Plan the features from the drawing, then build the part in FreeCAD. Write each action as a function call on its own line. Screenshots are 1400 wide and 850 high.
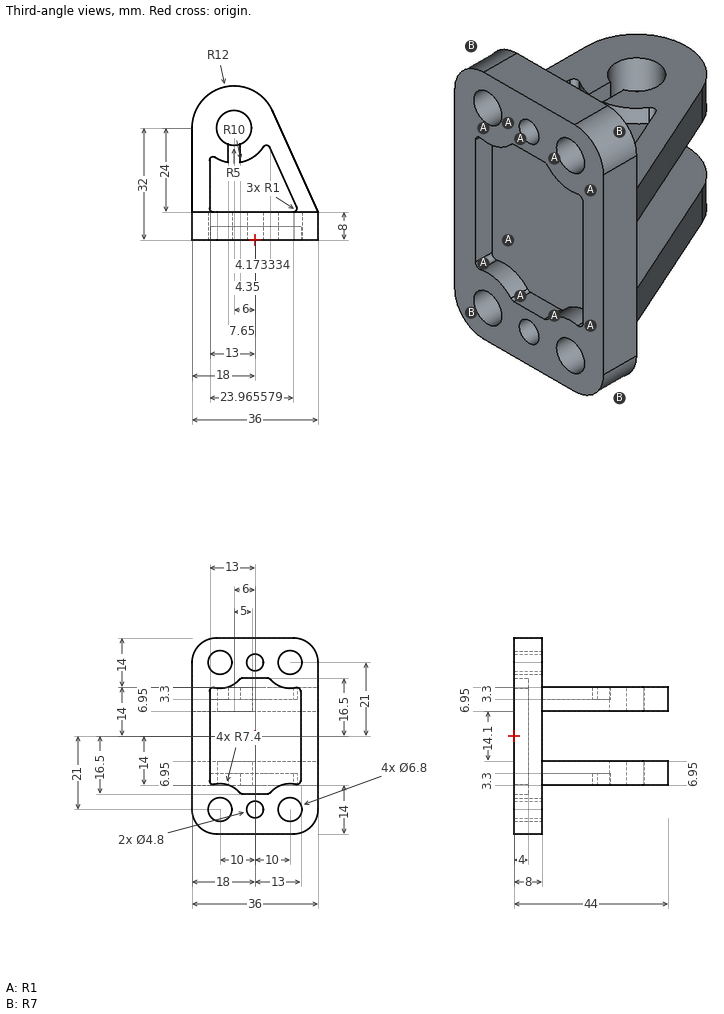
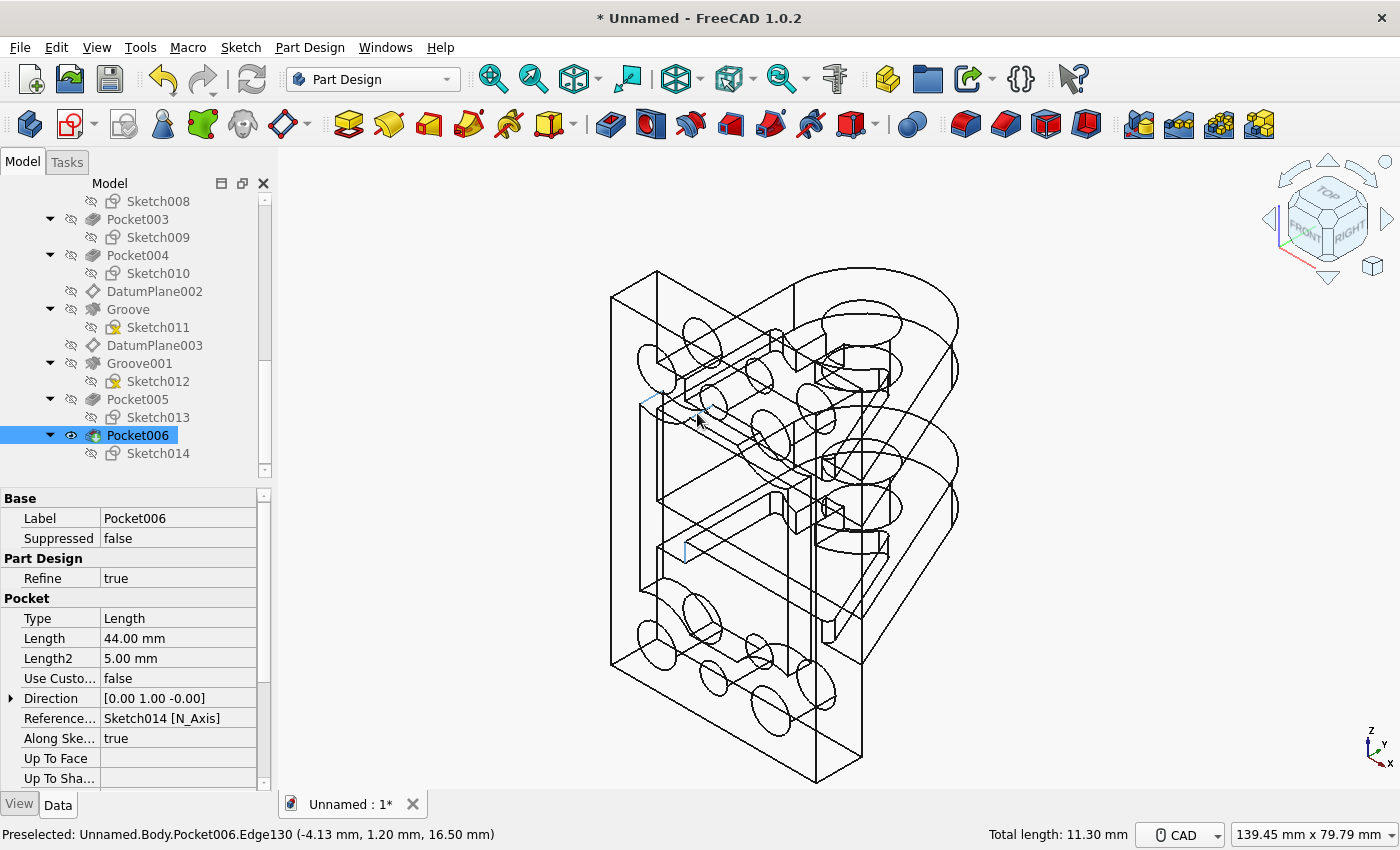
click(746, 439, ctrl)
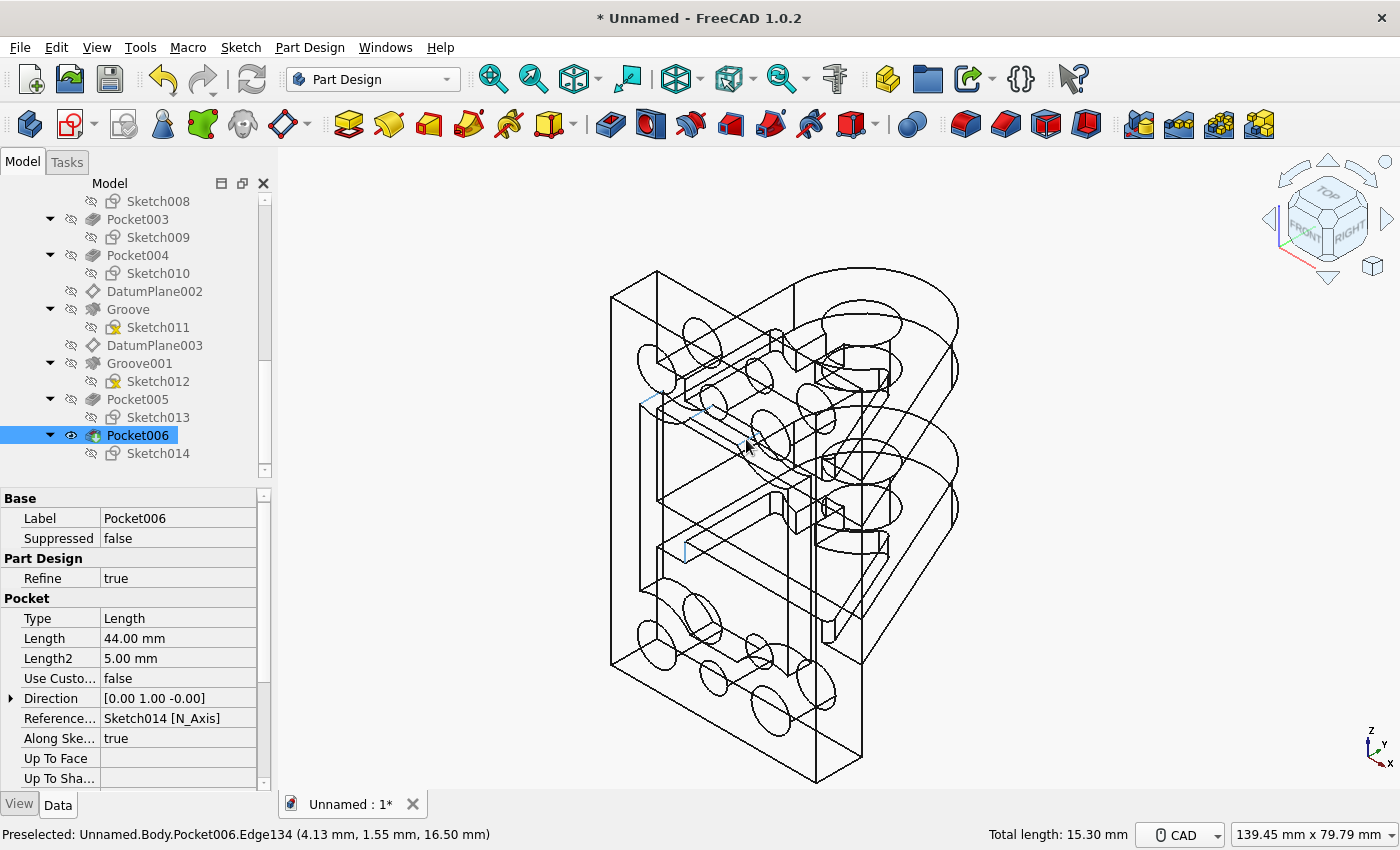
click(799, 482, ctrl)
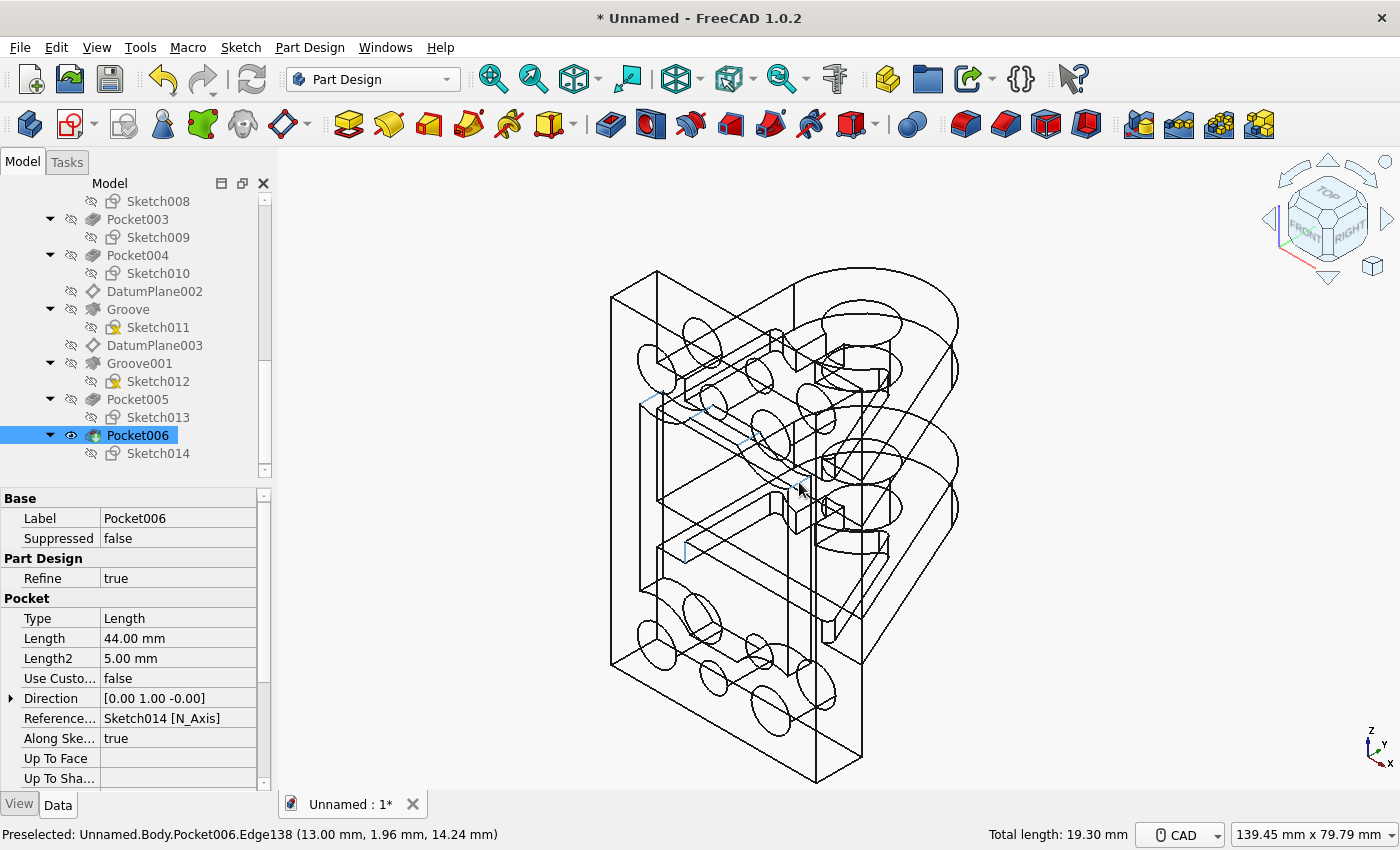
click(799, 669, ctrl)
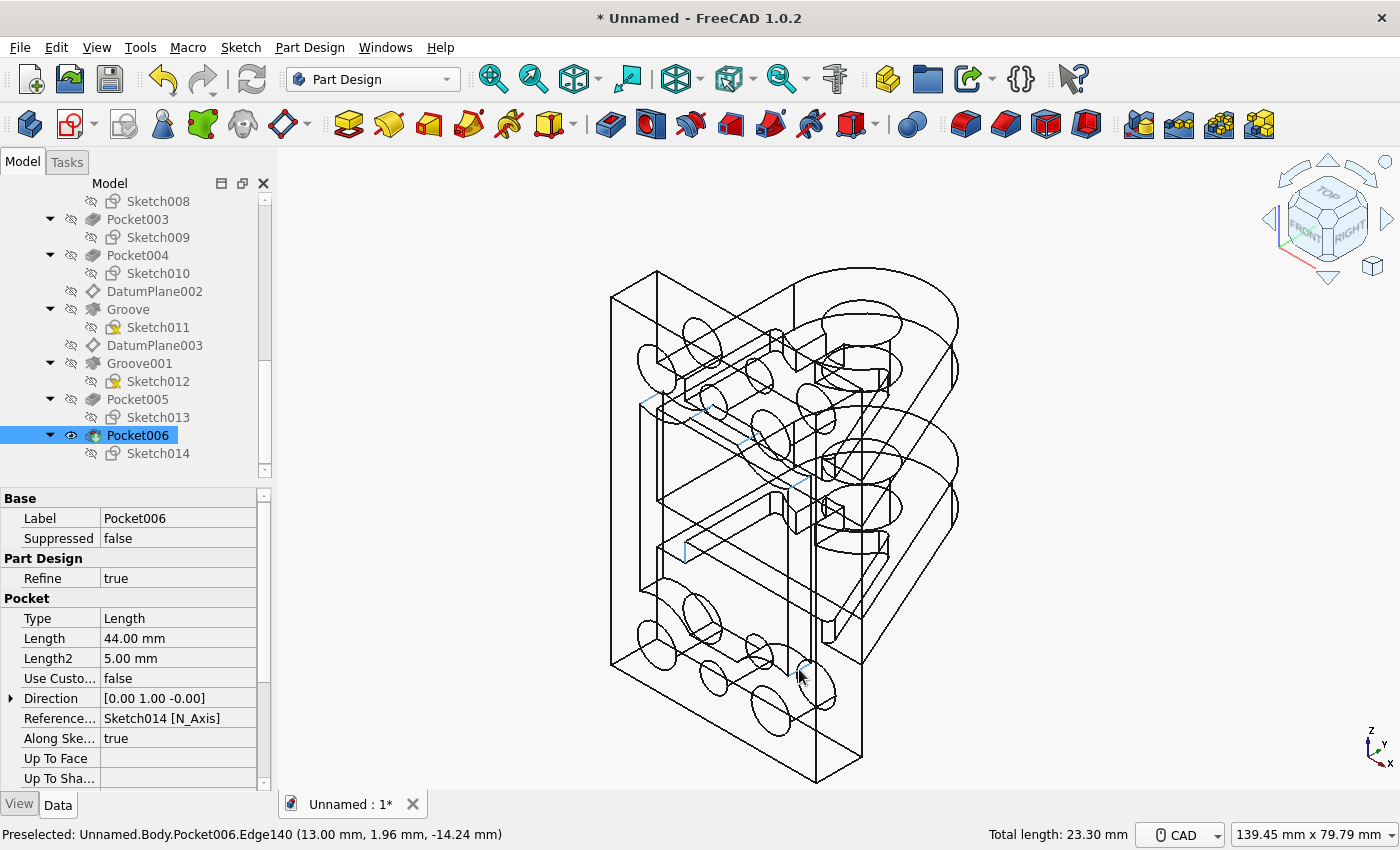
click(757, 650, ctrl)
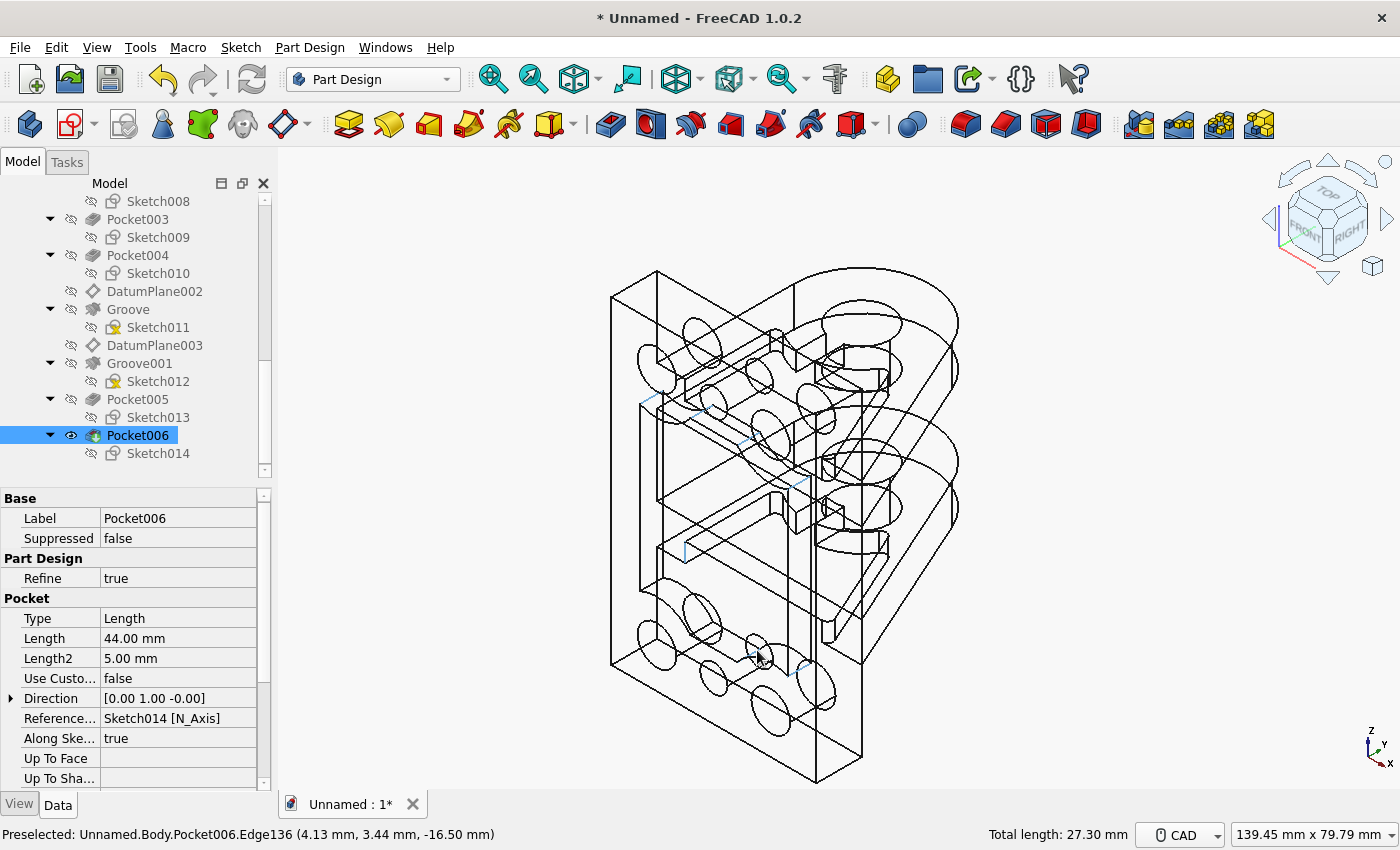
click(702, 628, ctrl)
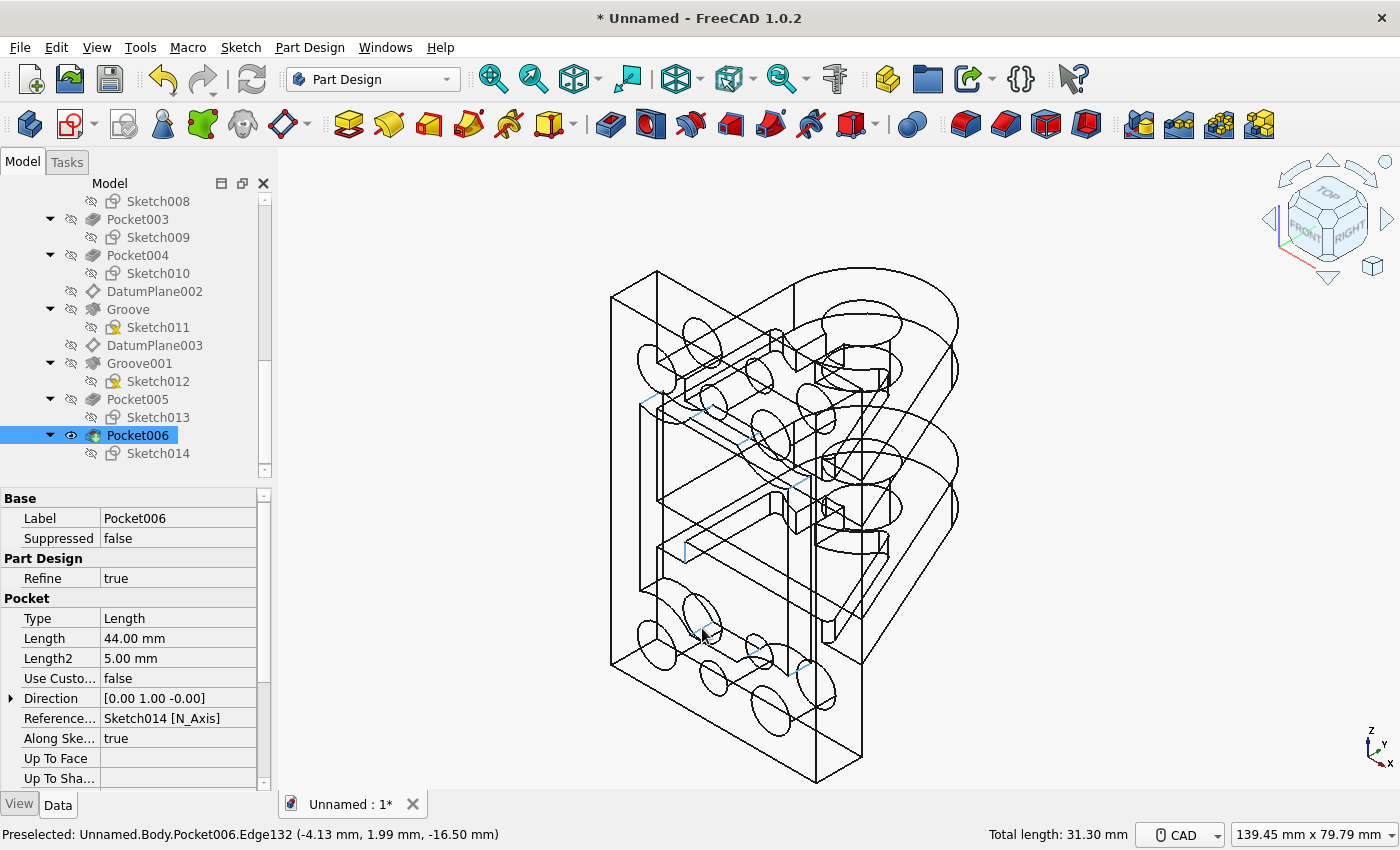
click(651, 583, ctrl)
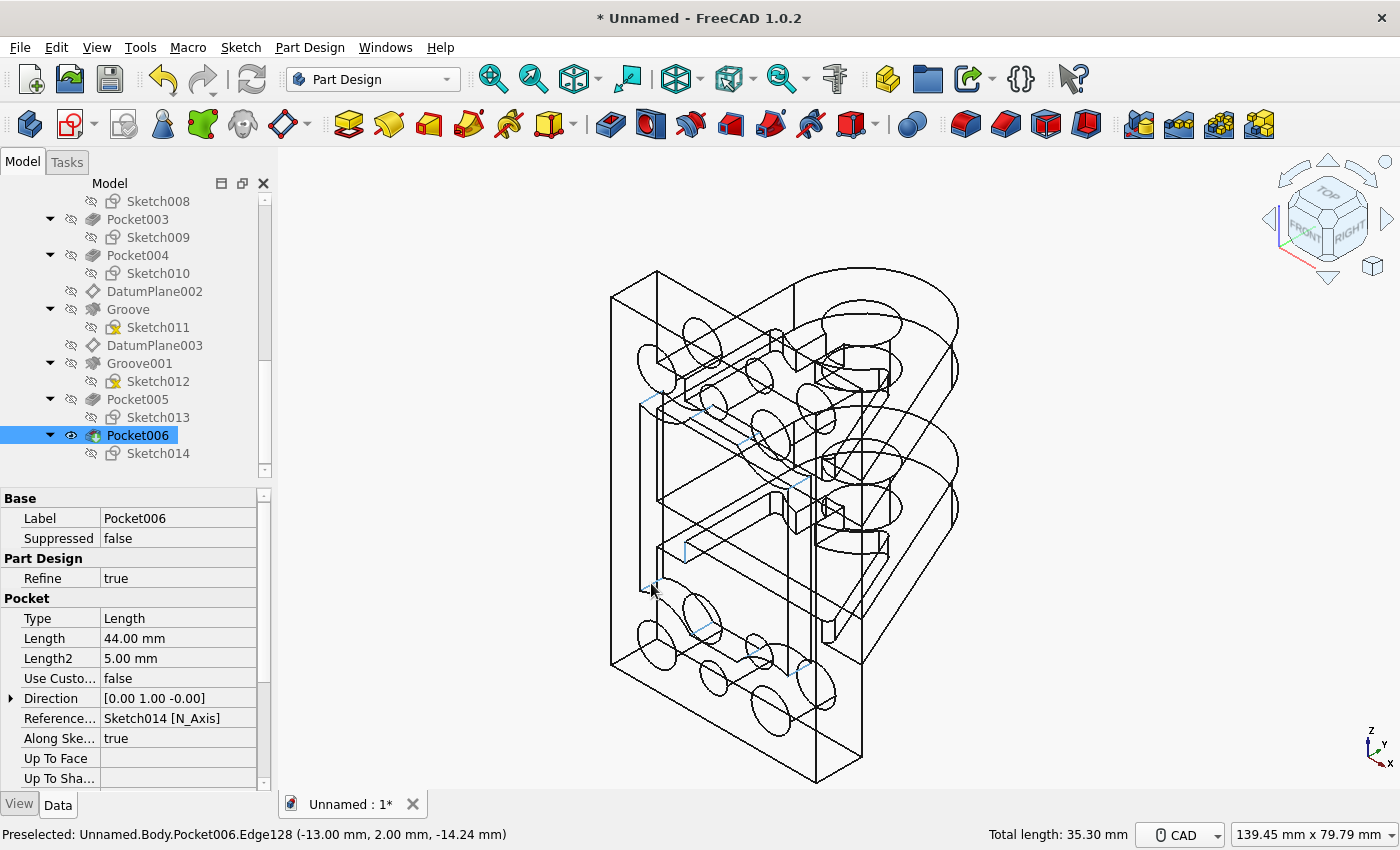
click(685, 389, ctrl)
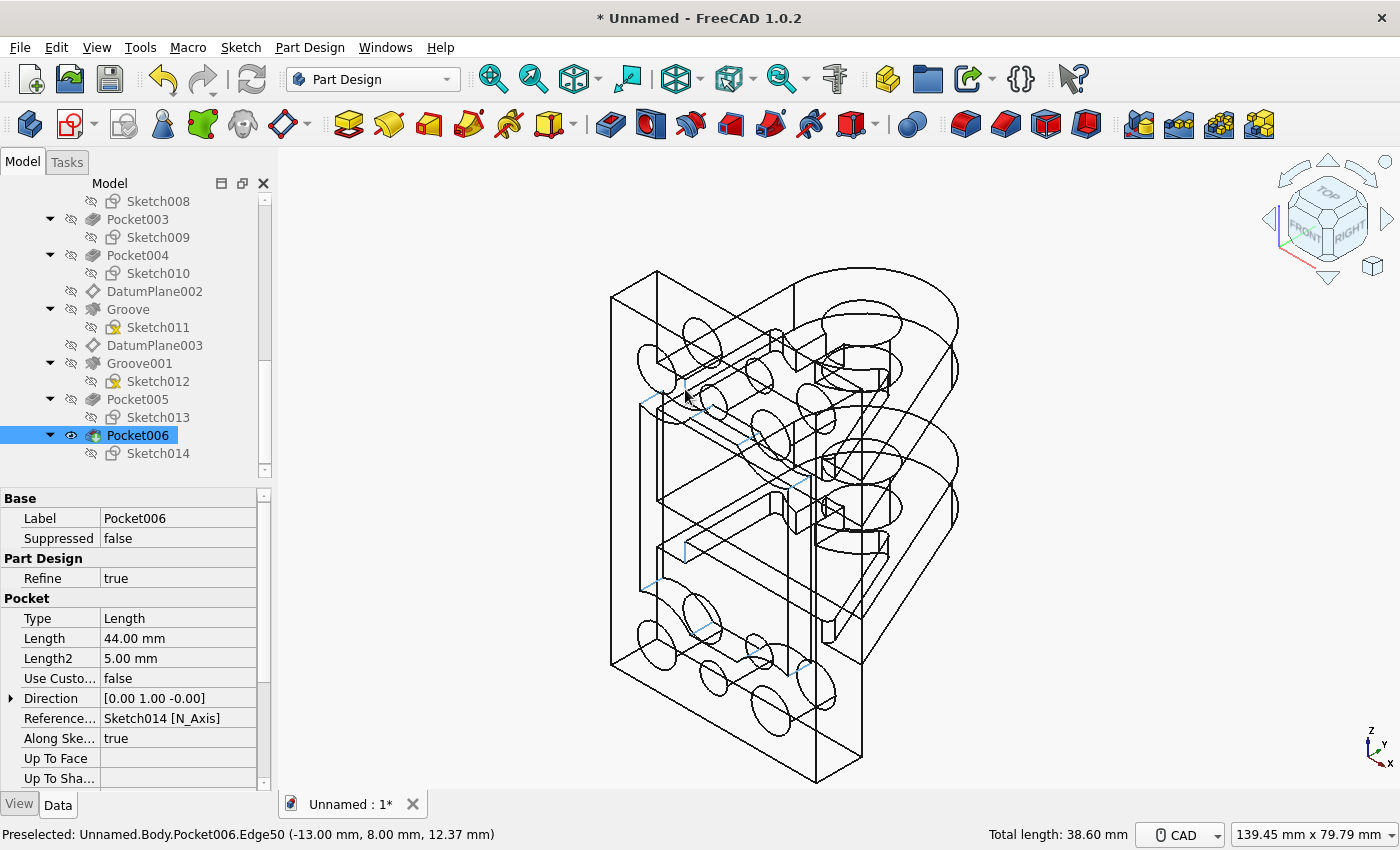
key(v)
key(1)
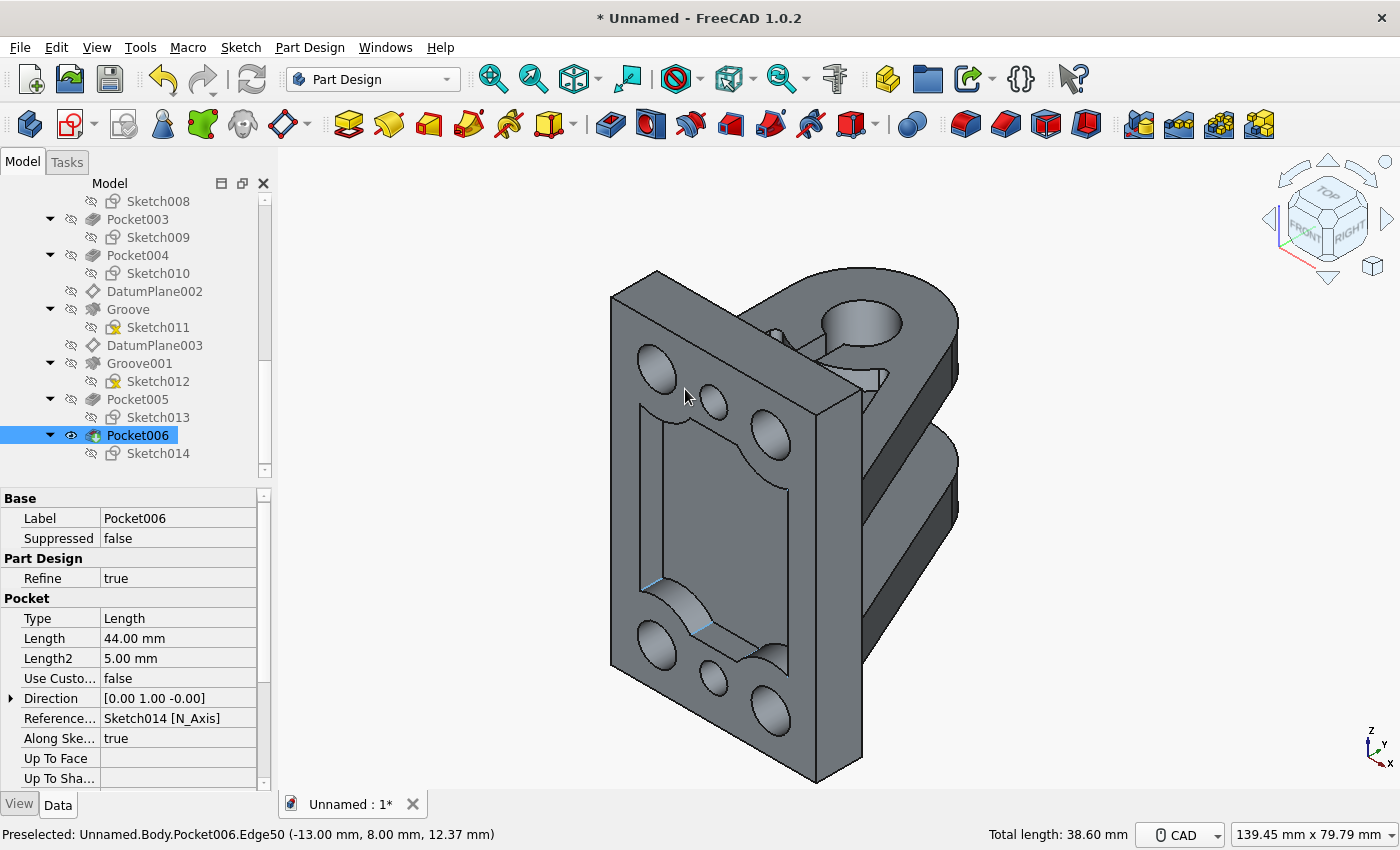
click(966, 124)